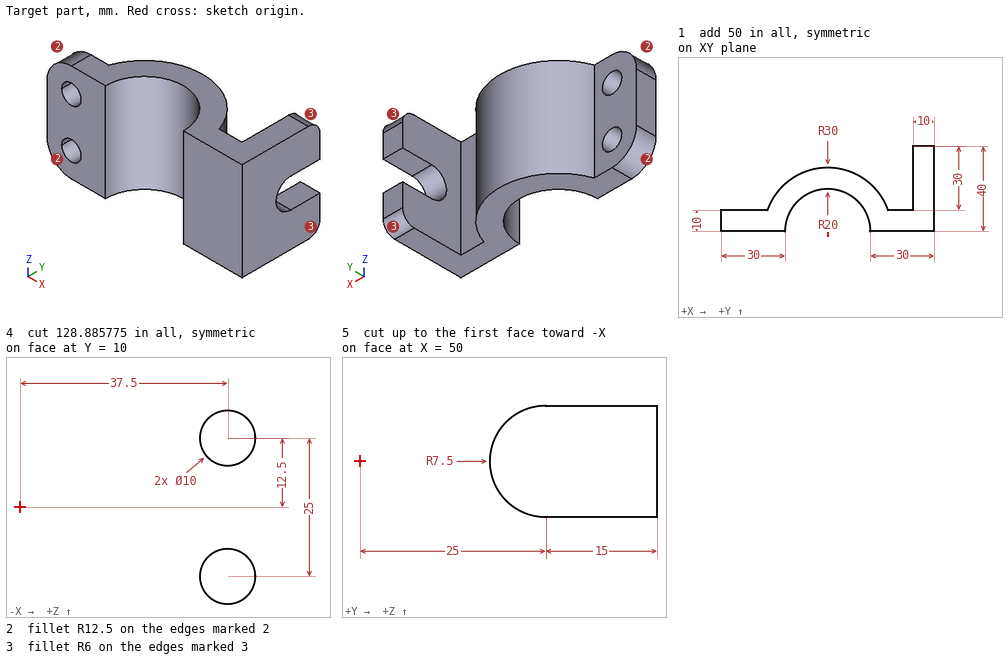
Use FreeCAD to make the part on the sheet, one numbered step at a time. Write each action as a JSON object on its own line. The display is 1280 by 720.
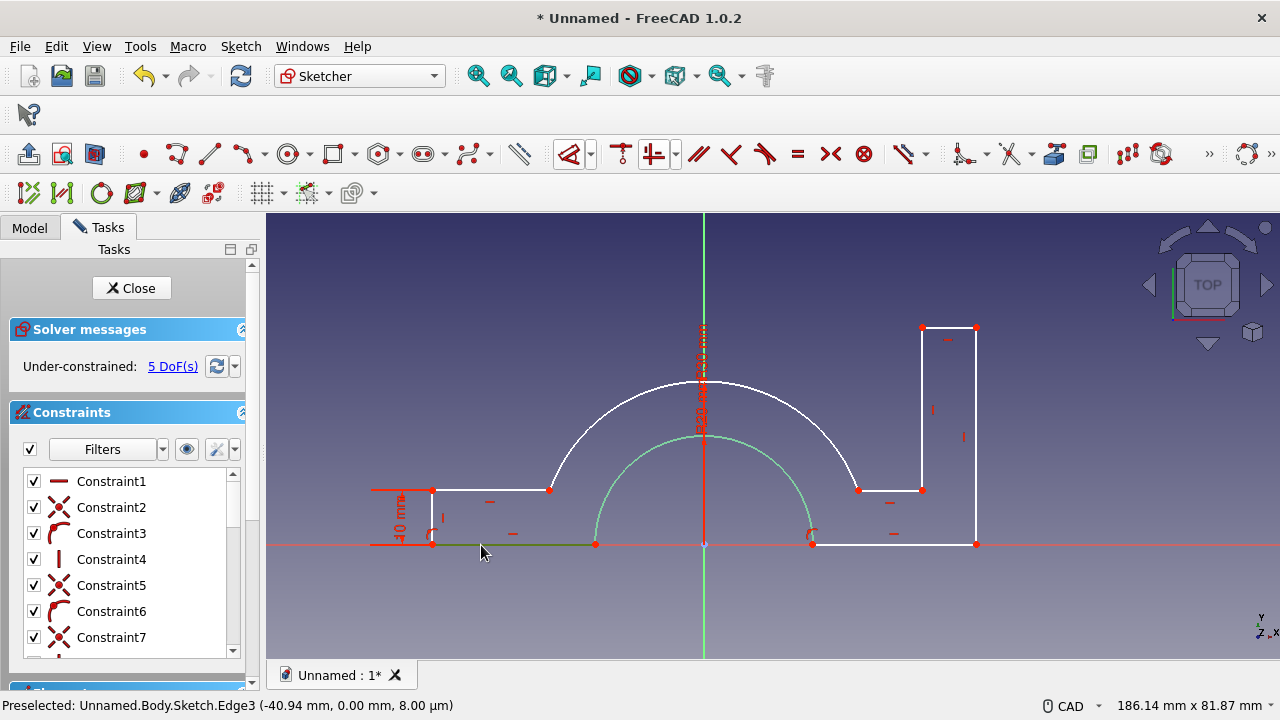
{"action": "key", "text": "l"}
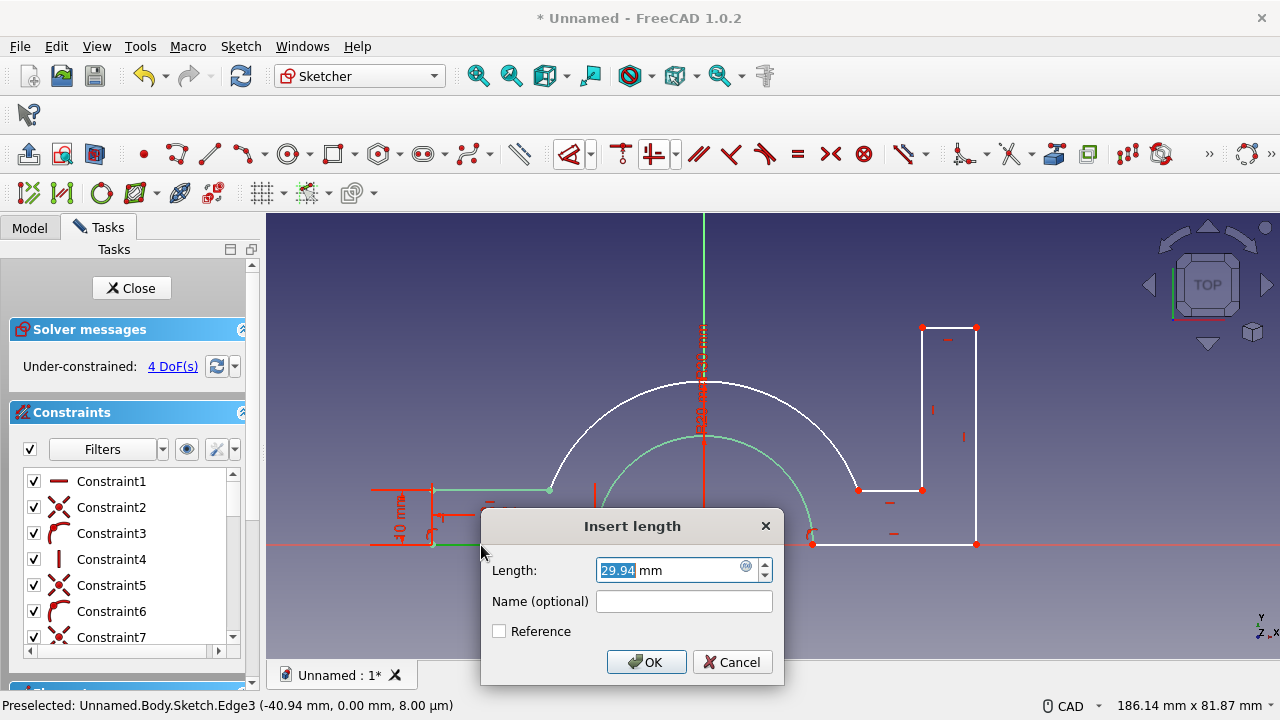
{"action": "type", "text": "30"}
{"action": "key", "text": "Return"}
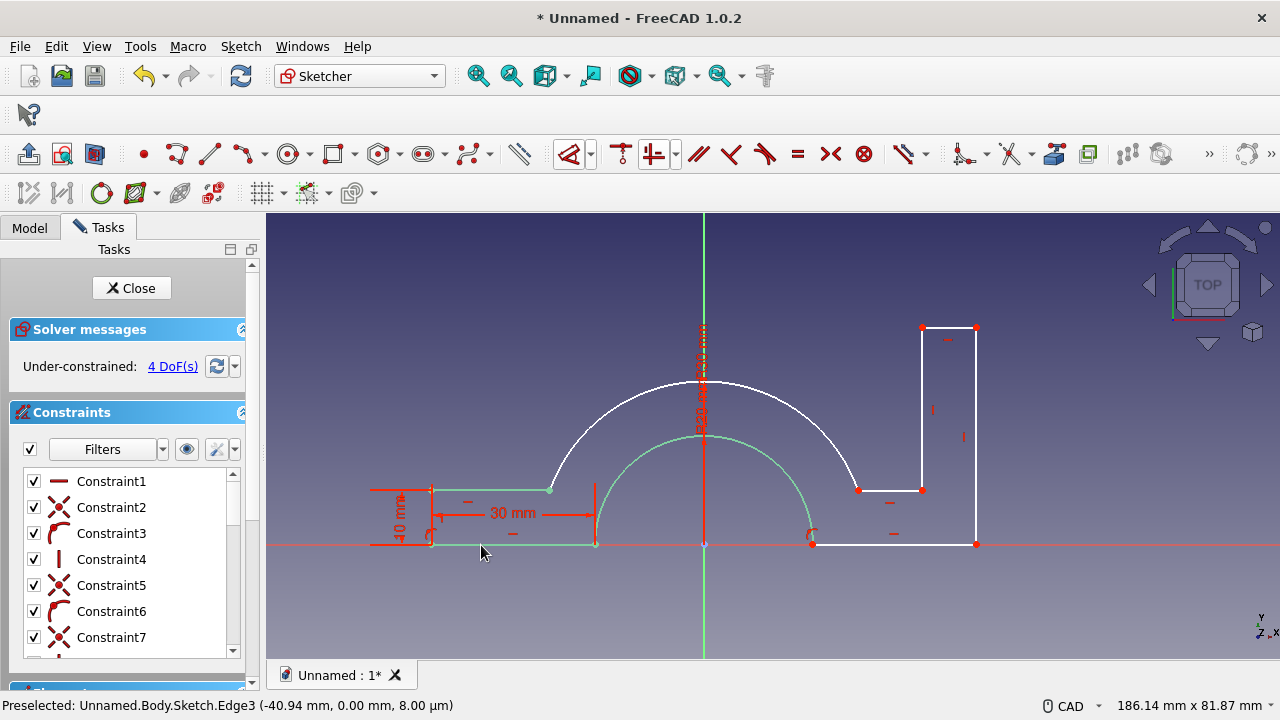
{"action": "left_click", "coordinate": [862, 545]}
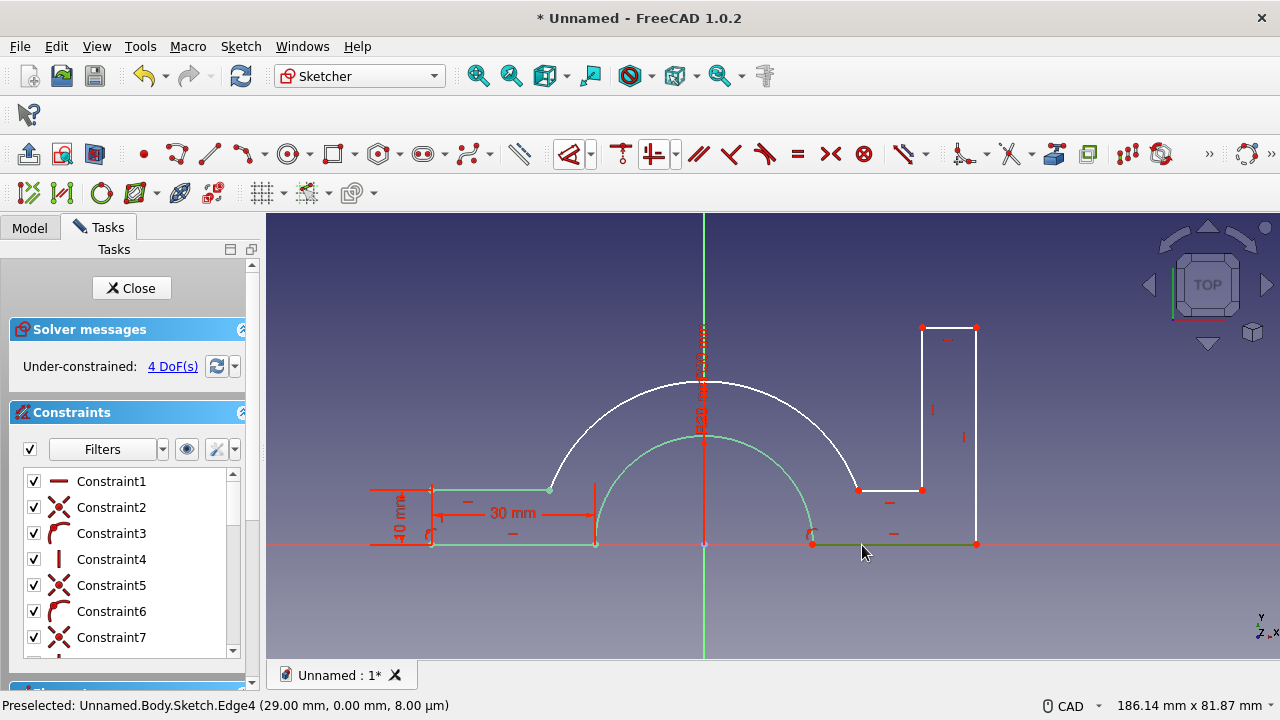
{"action": "left_click", "coordinate": [590, 154]}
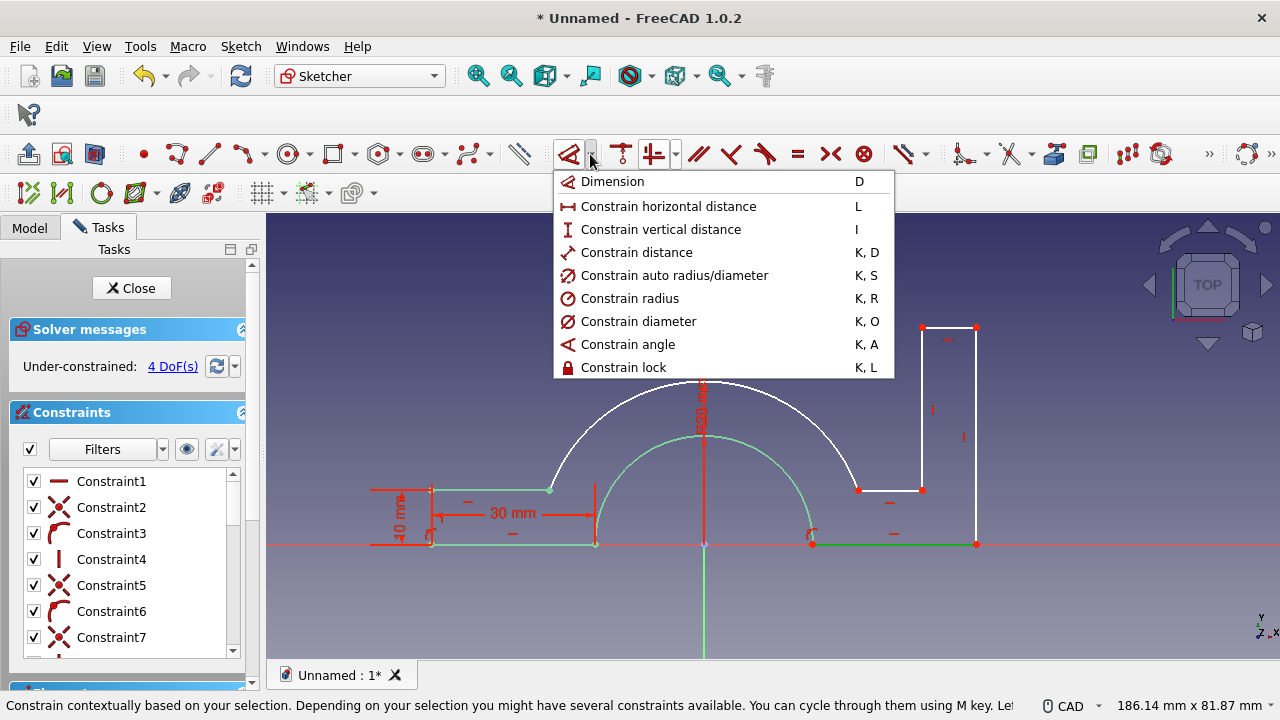
{"action": "left_click", "coordinate": [724, 206]}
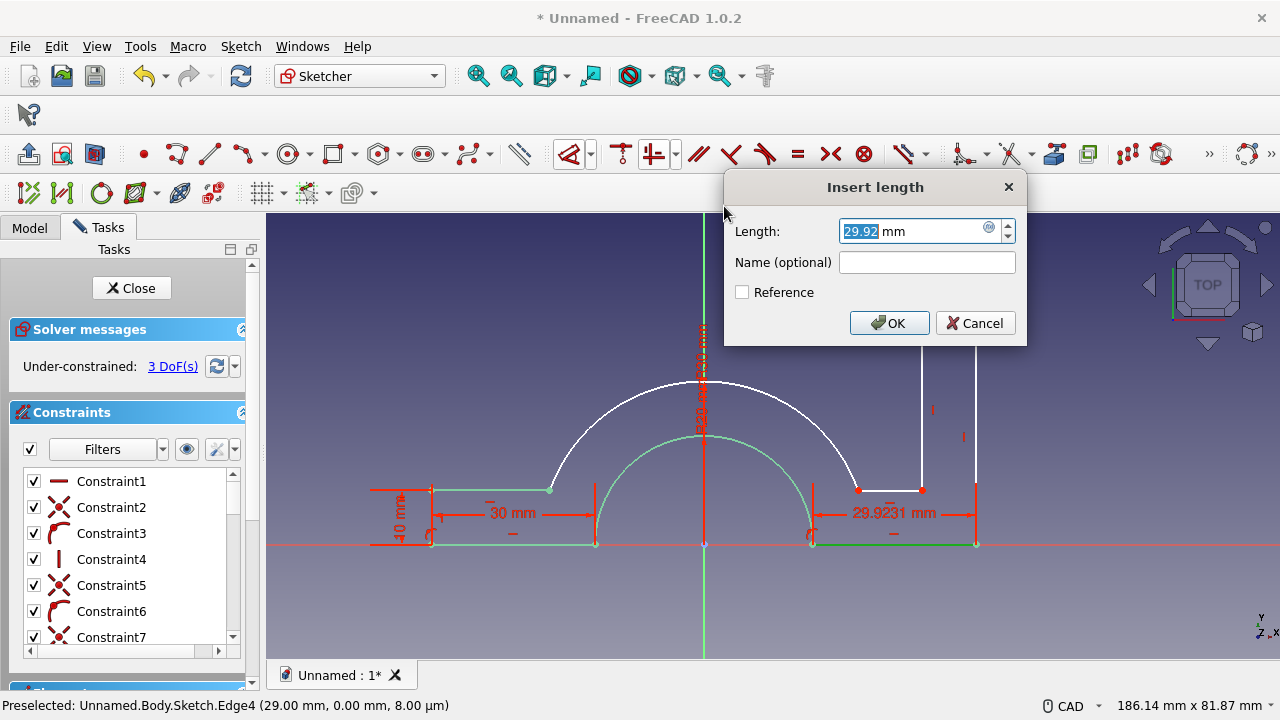
{"action": "type", "text": "30"}
{"action": "key", "text": "Return"}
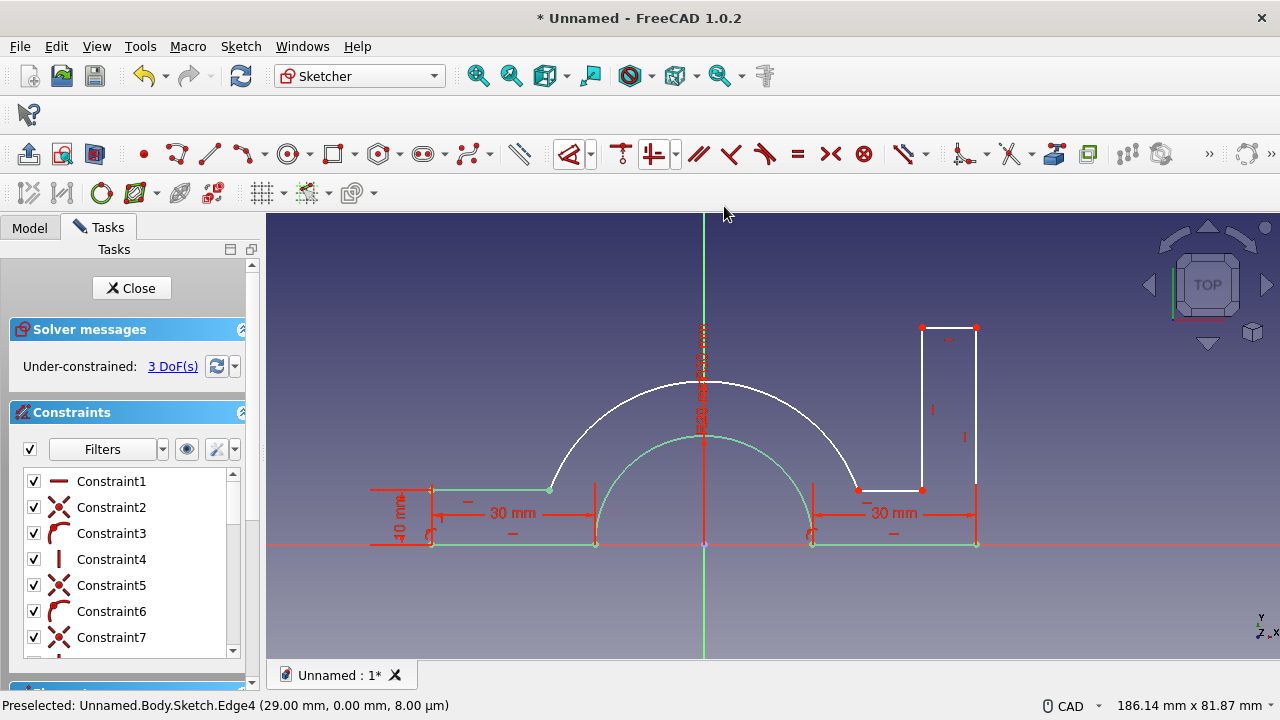
{"action": "left_click", "coordinate": [976, 480]}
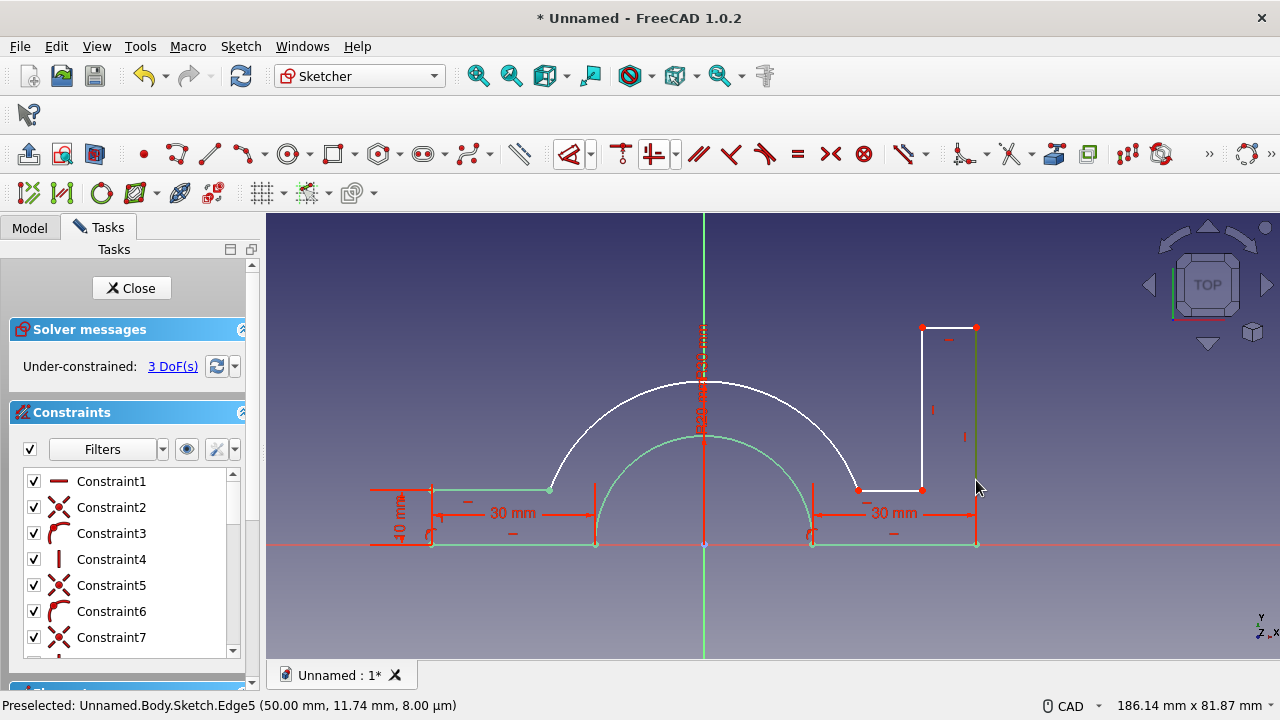
{"action": "left_click", "coordinate": [590, 154]}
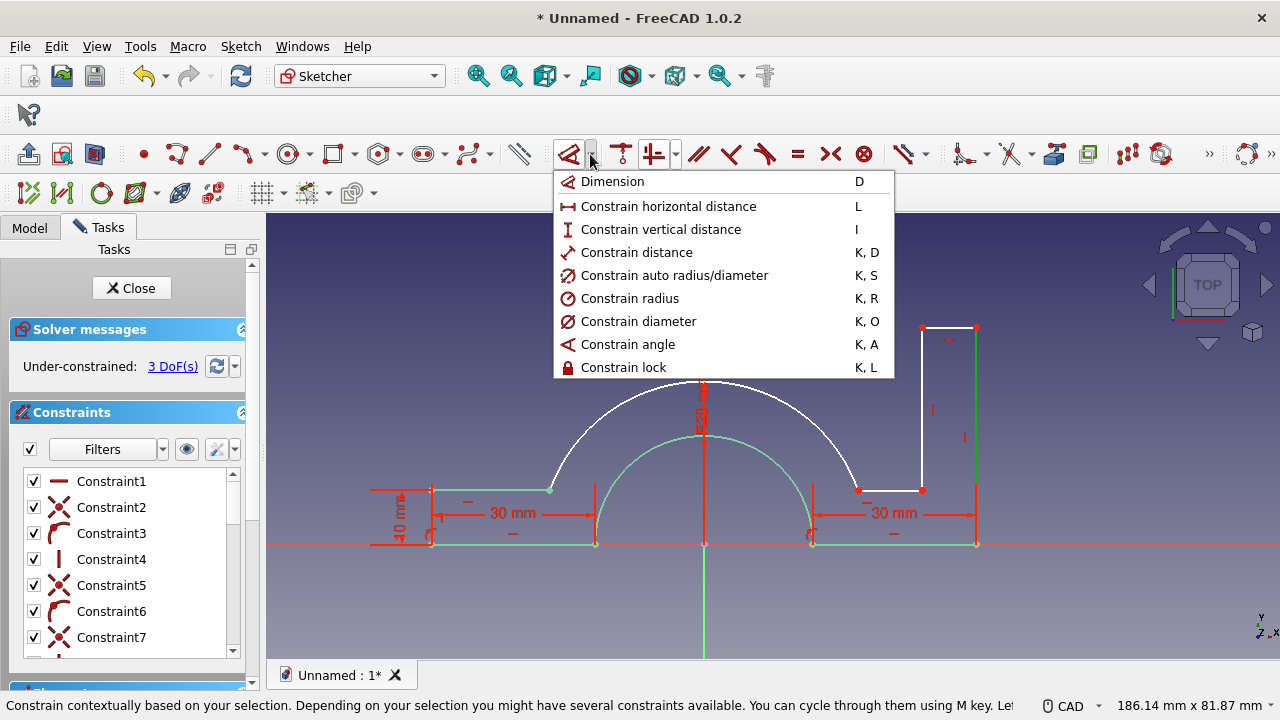
{"action": "left_click", "coordinate": [724, 230]}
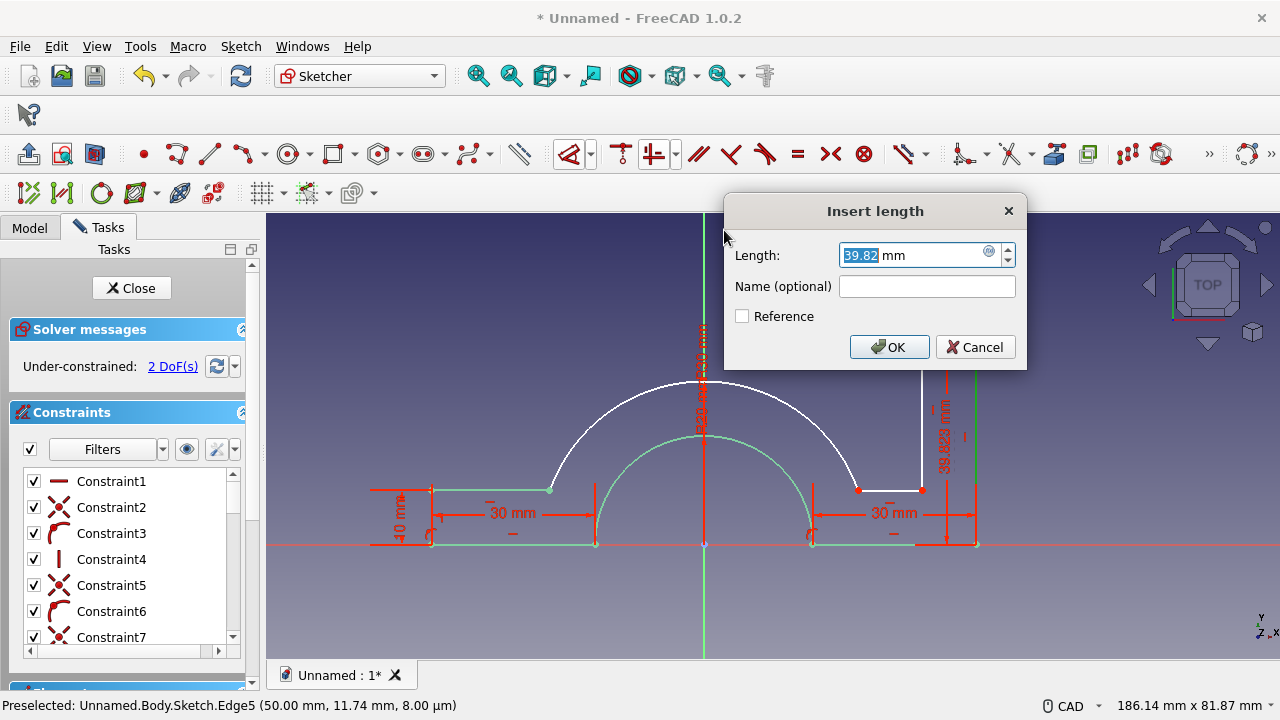
{"action": "type", "text": "40"}
{"action": "key", "text": "Return"}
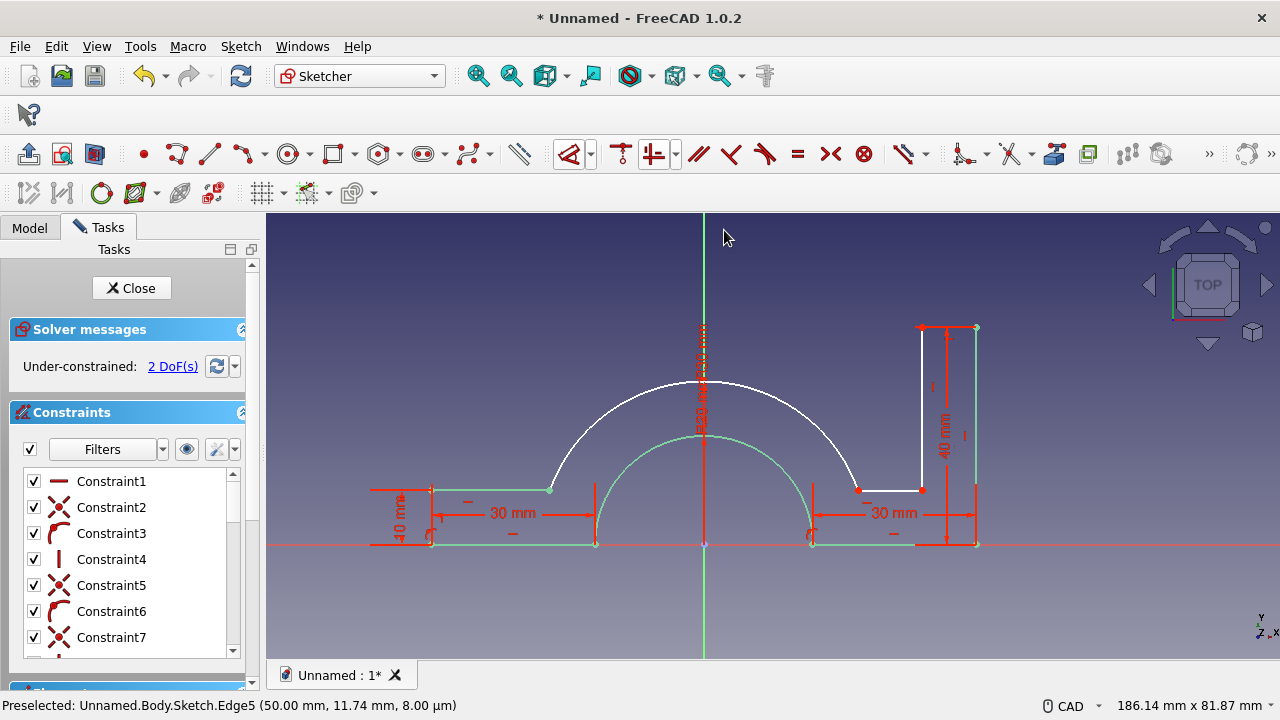
{"action": "left_click", "coordinate": [960, 327]}